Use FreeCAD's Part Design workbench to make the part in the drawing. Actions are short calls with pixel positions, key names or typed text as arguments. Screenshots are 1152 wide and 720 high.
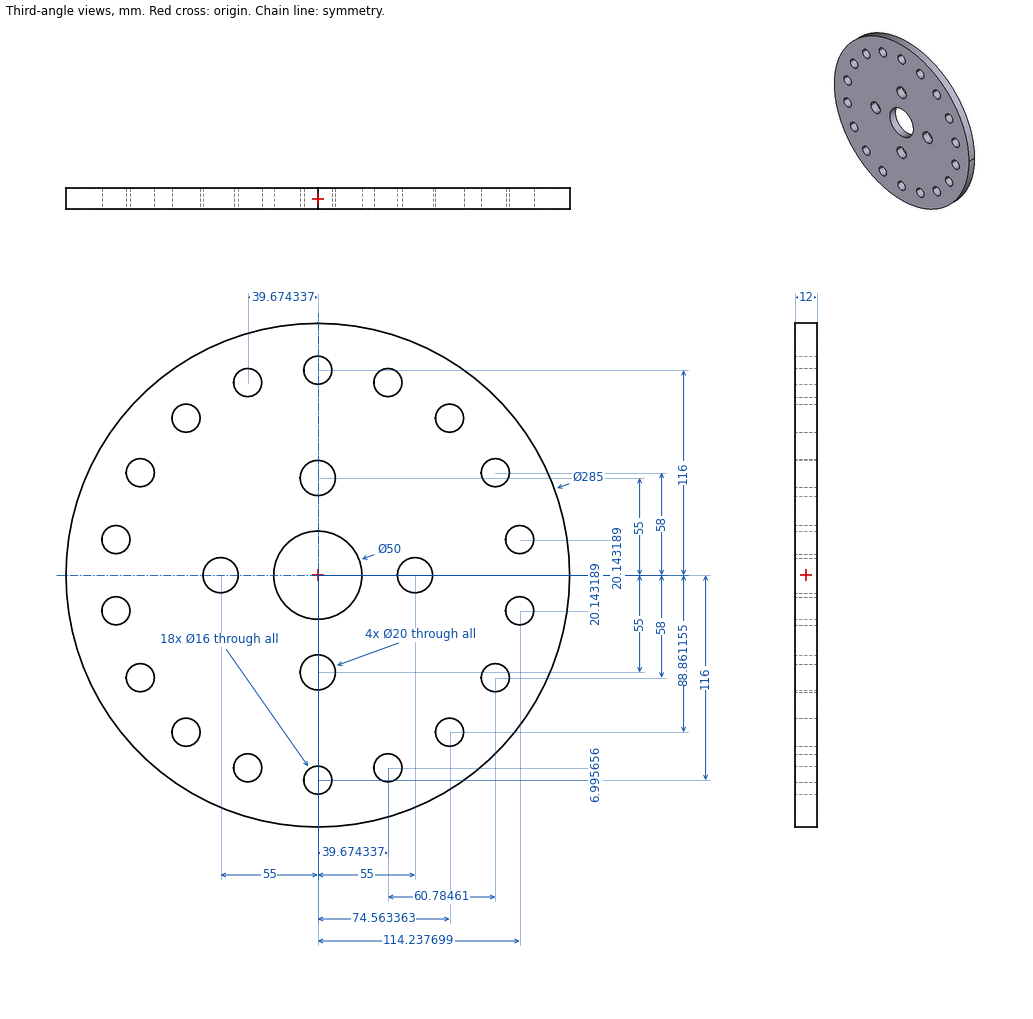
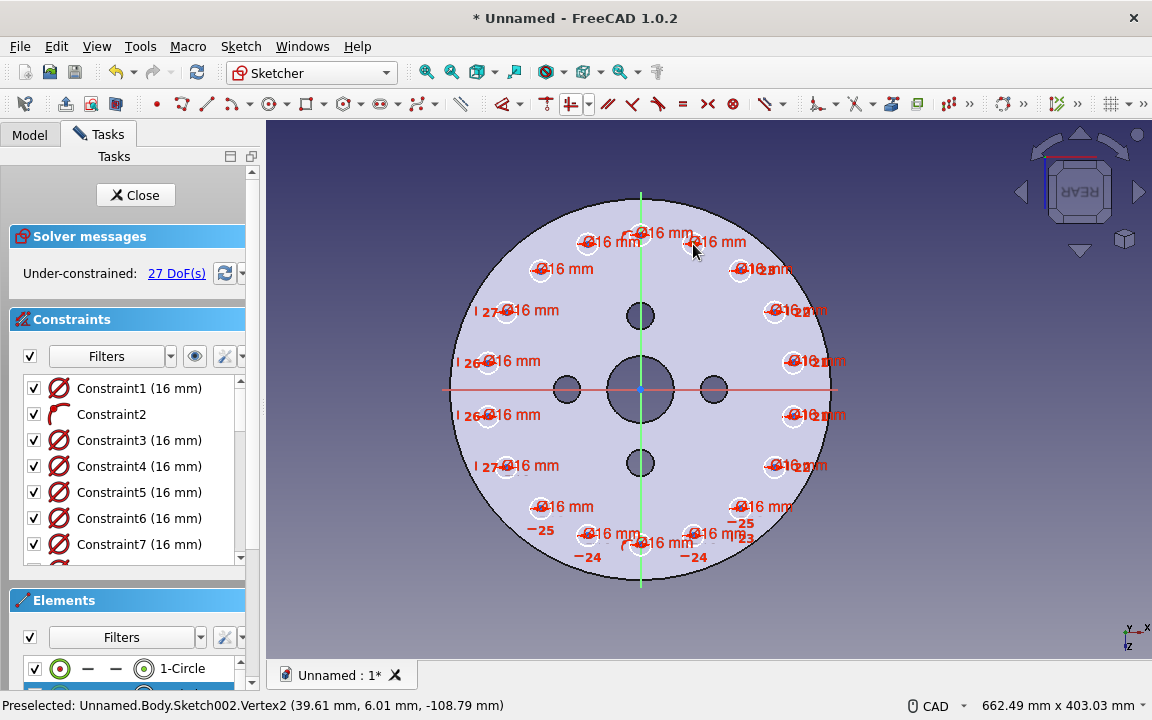
click(588, 244)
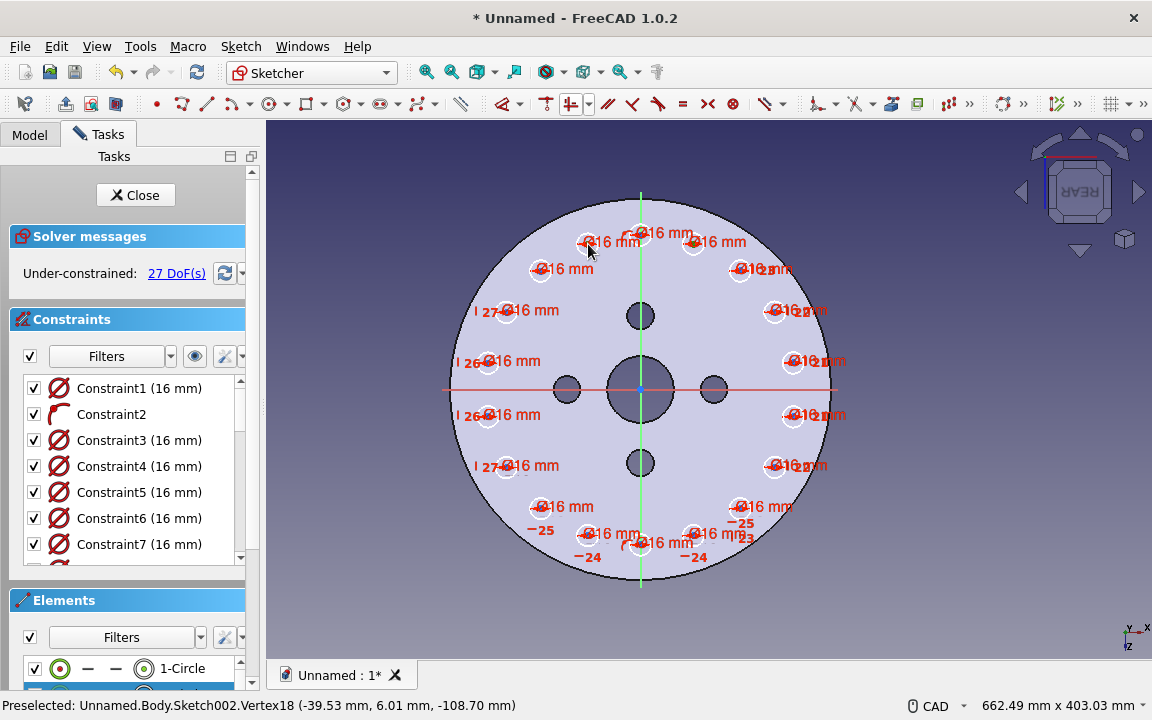
click(588, 104)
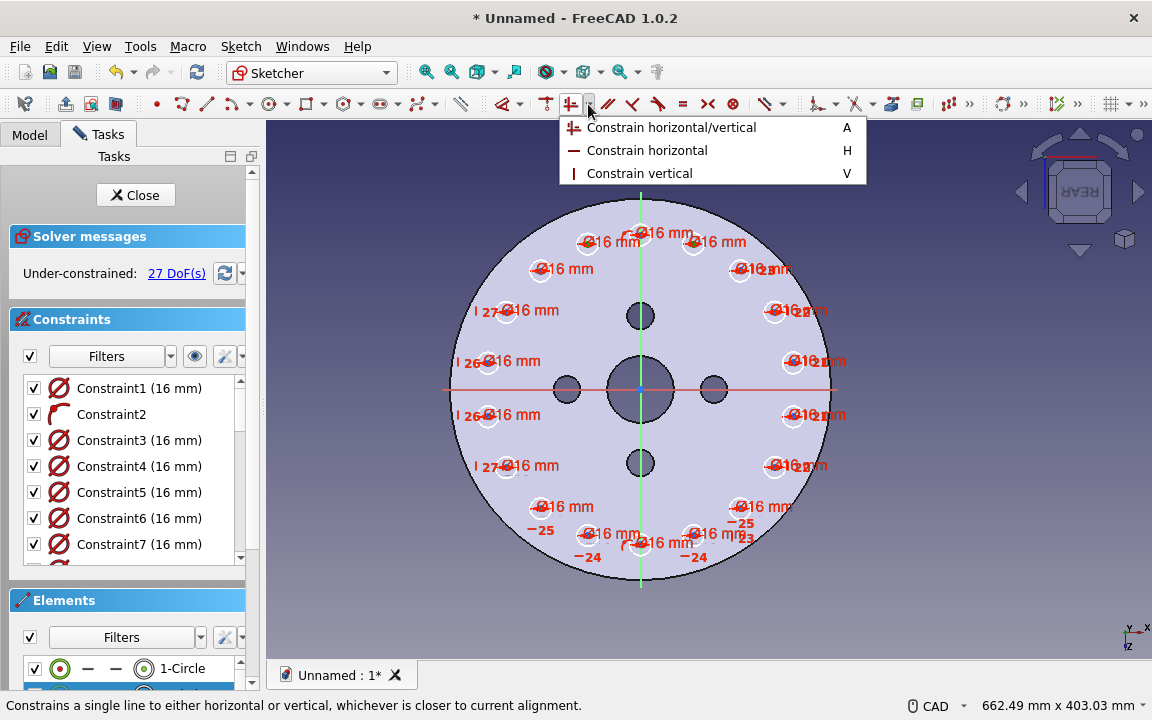
click(713, 150)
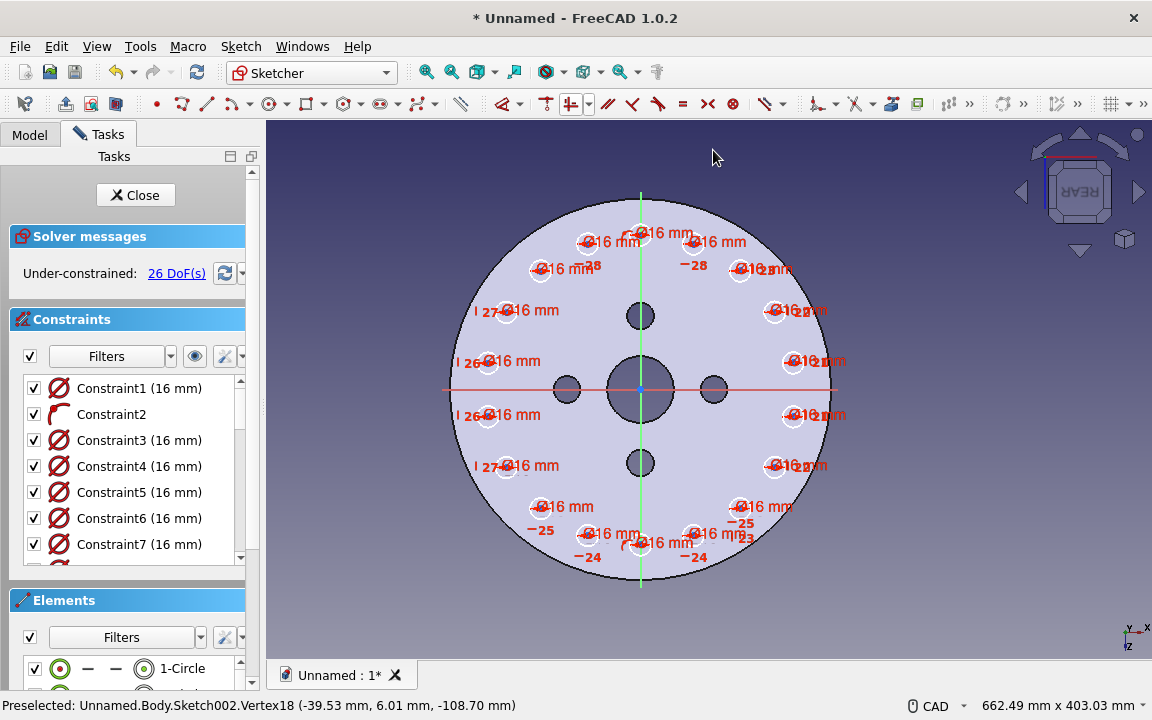
click(693, 244)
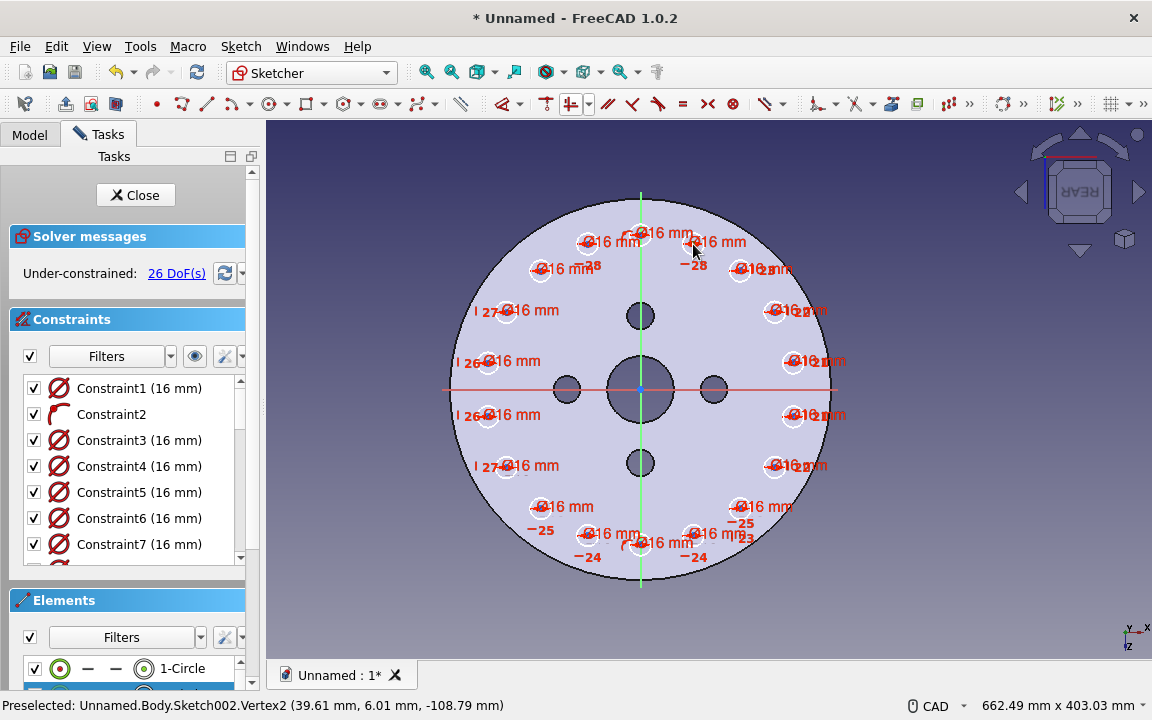
click(693, 536)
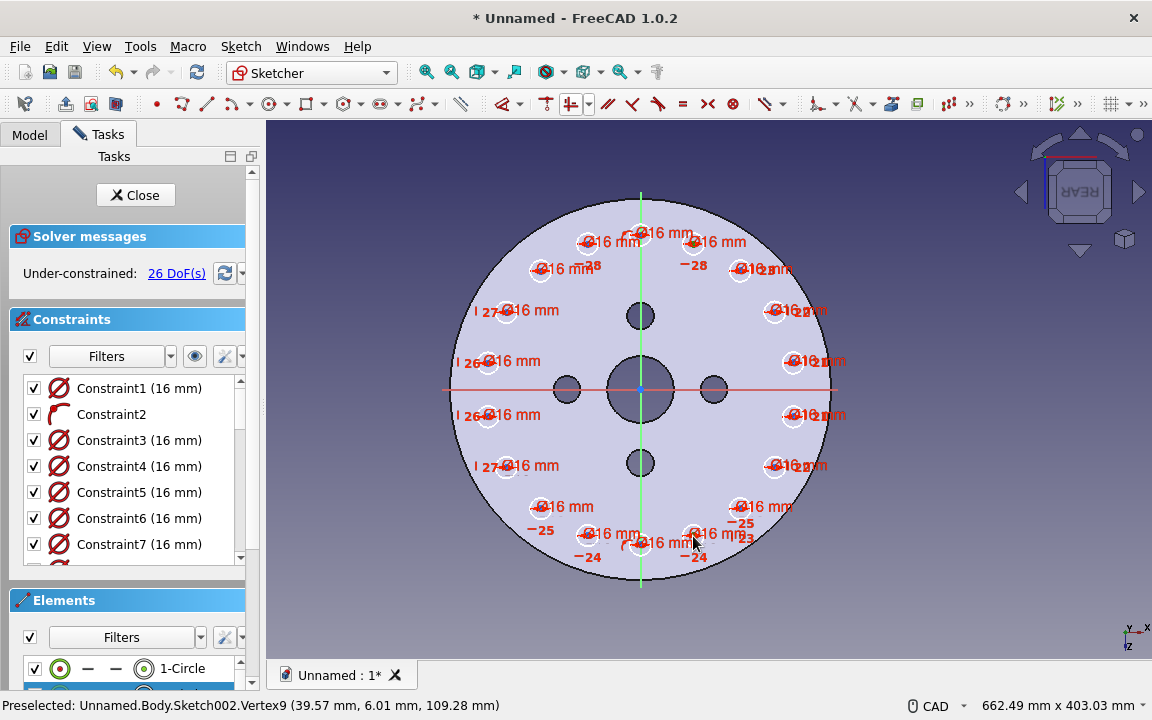
click(442, 389)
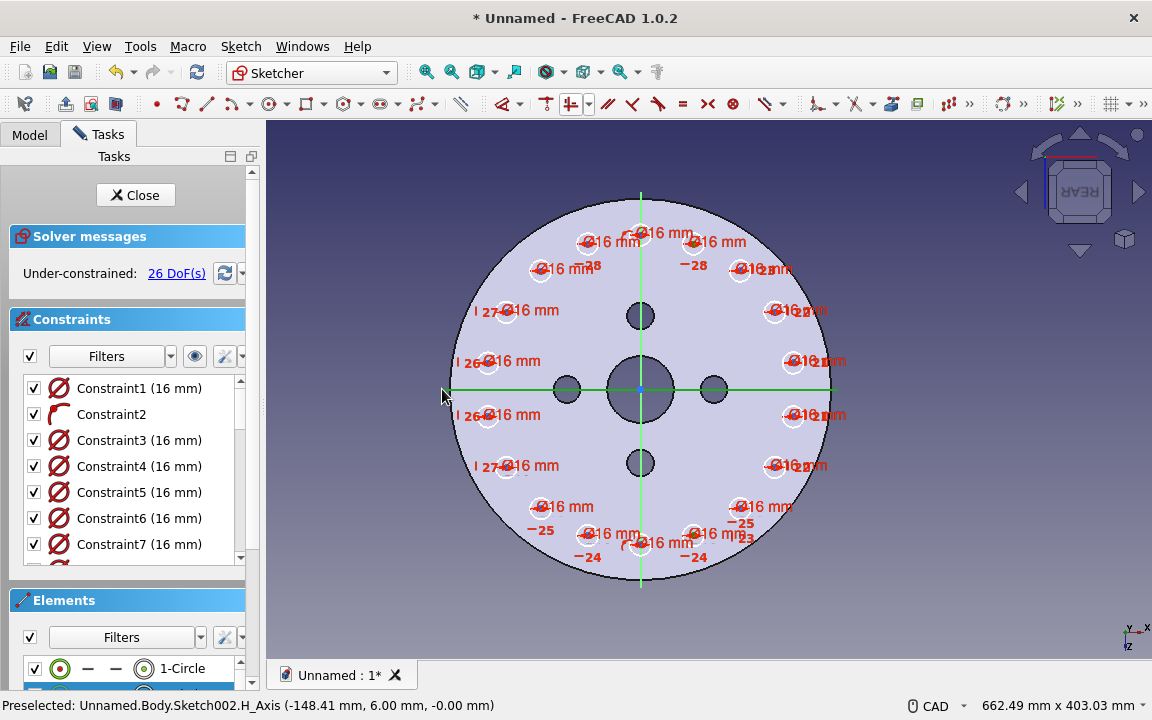
click(708, 104)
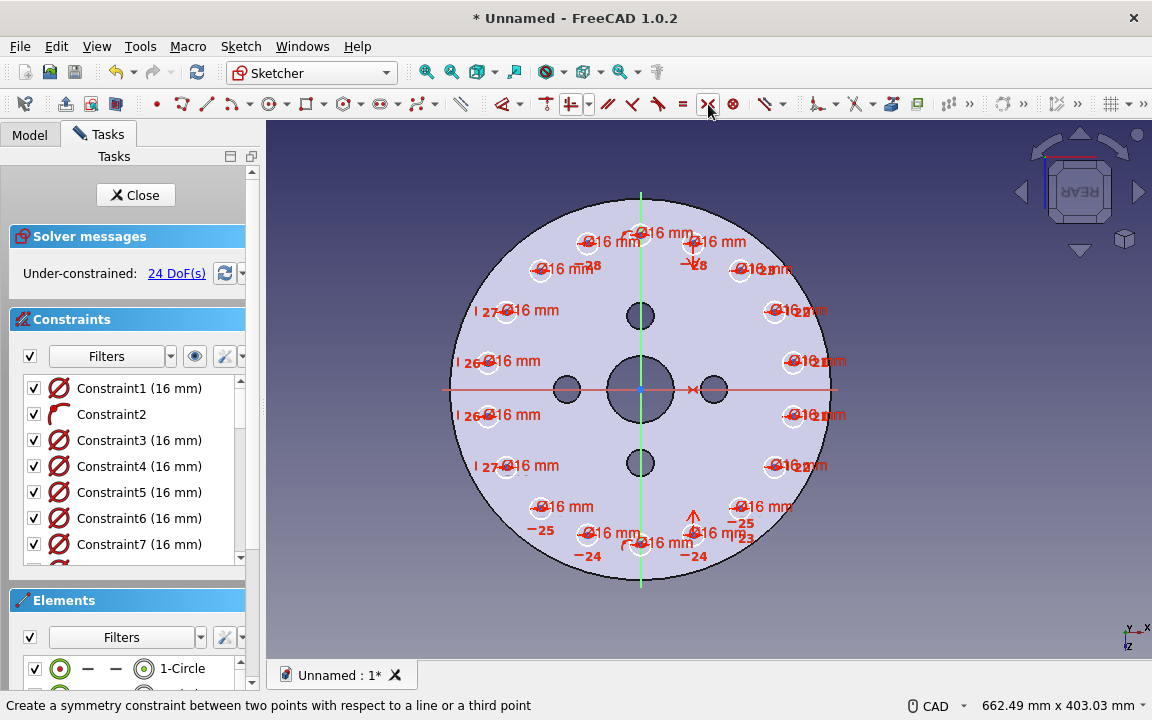
click(775, 467)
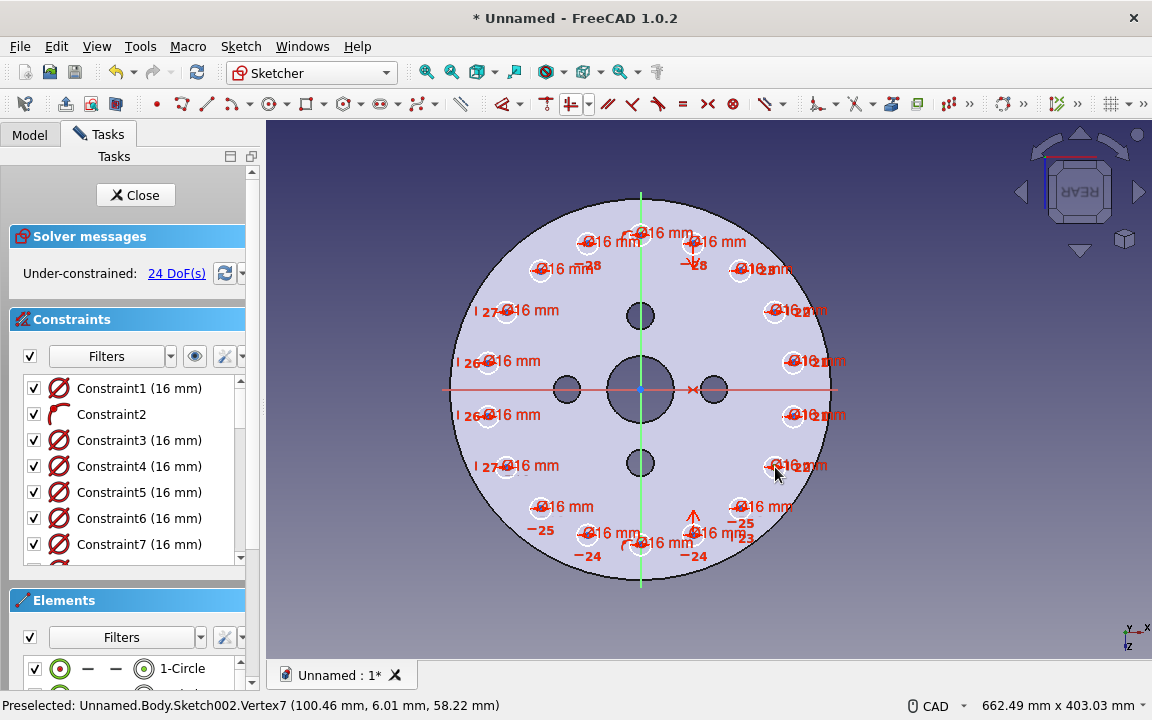
click(506, 468)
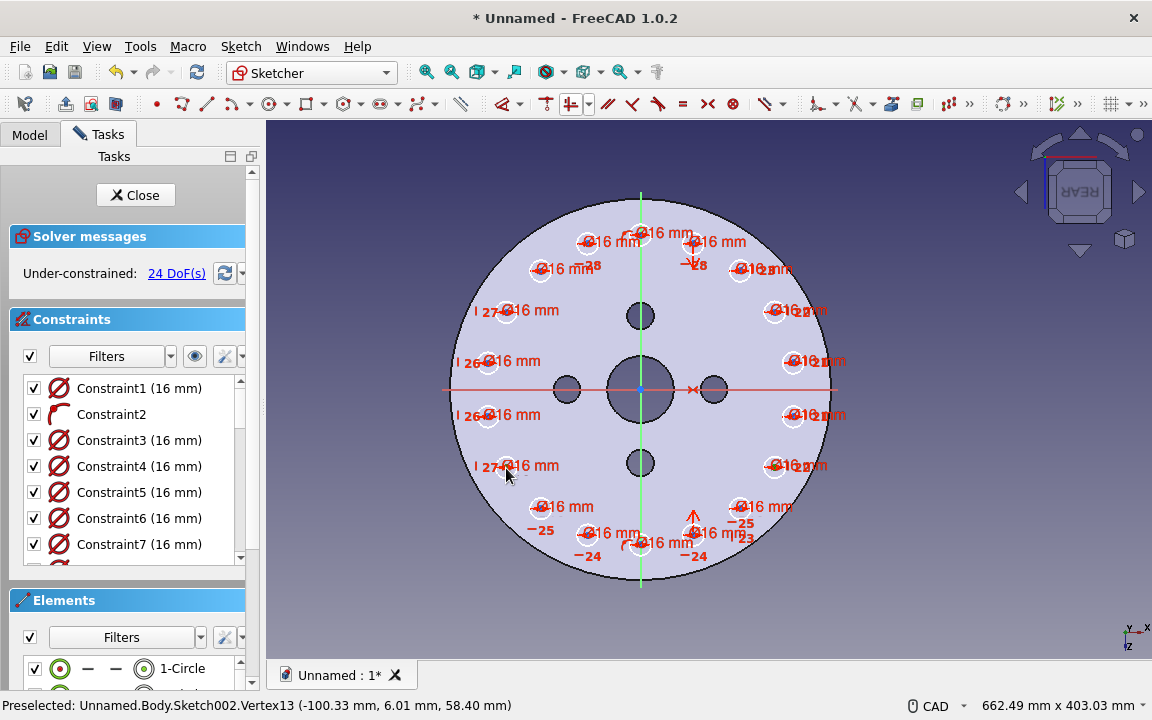
click(641, 493)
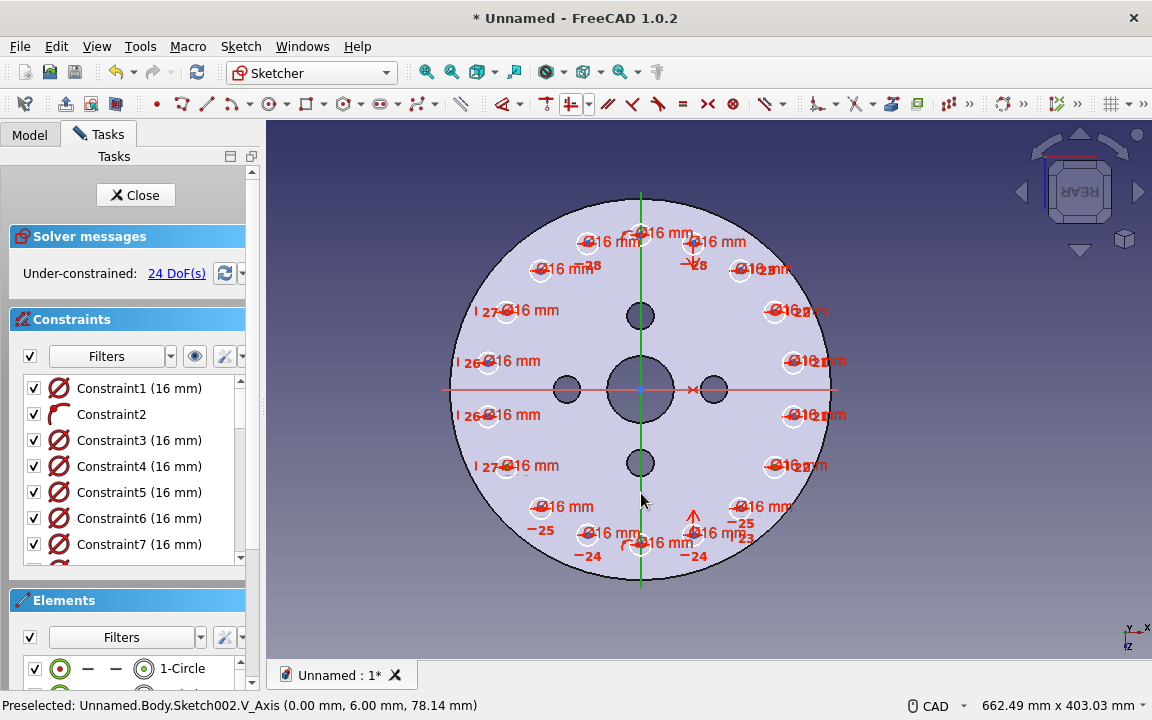
click(708, 104)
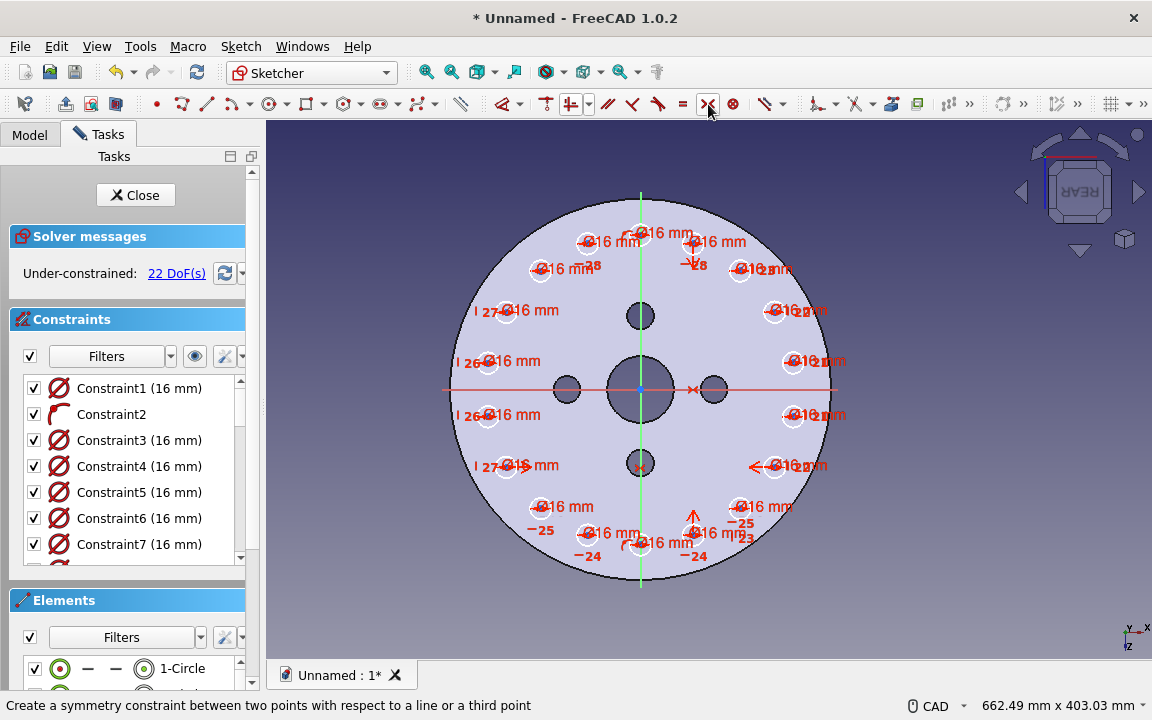
click(793, 417)